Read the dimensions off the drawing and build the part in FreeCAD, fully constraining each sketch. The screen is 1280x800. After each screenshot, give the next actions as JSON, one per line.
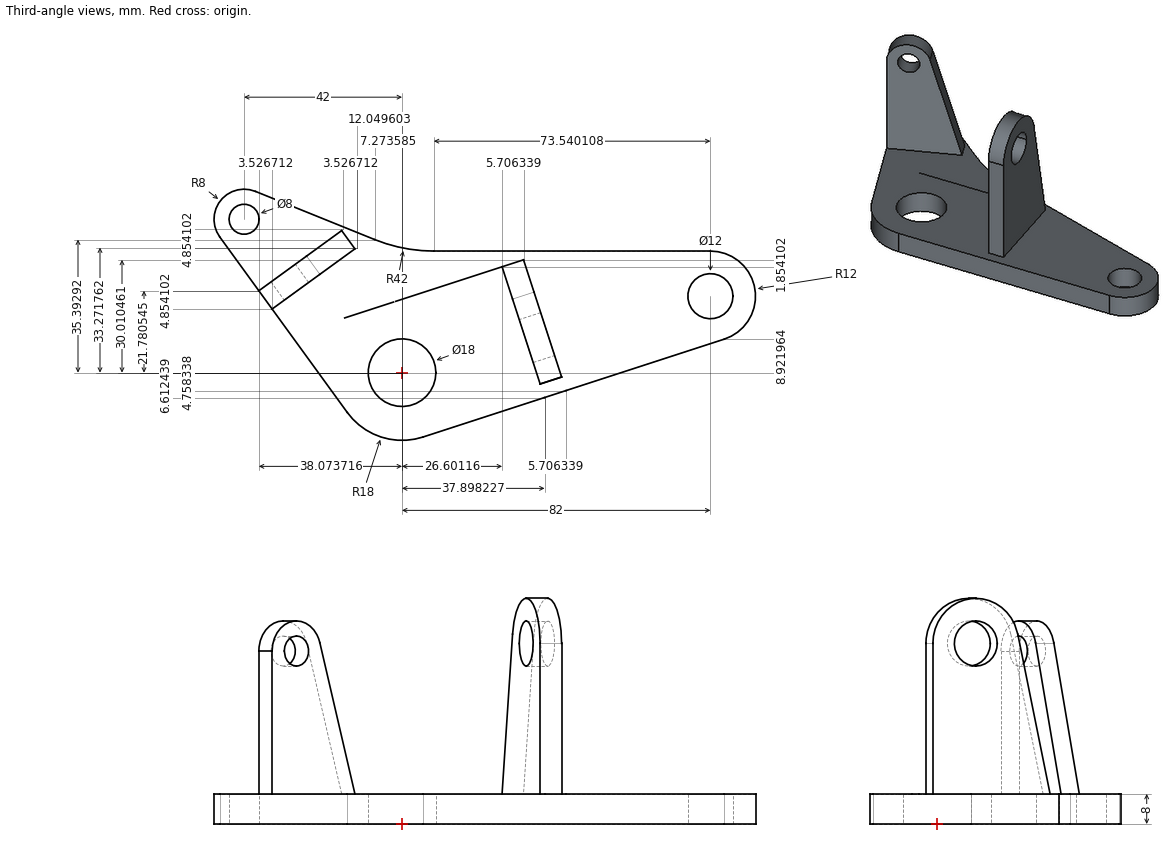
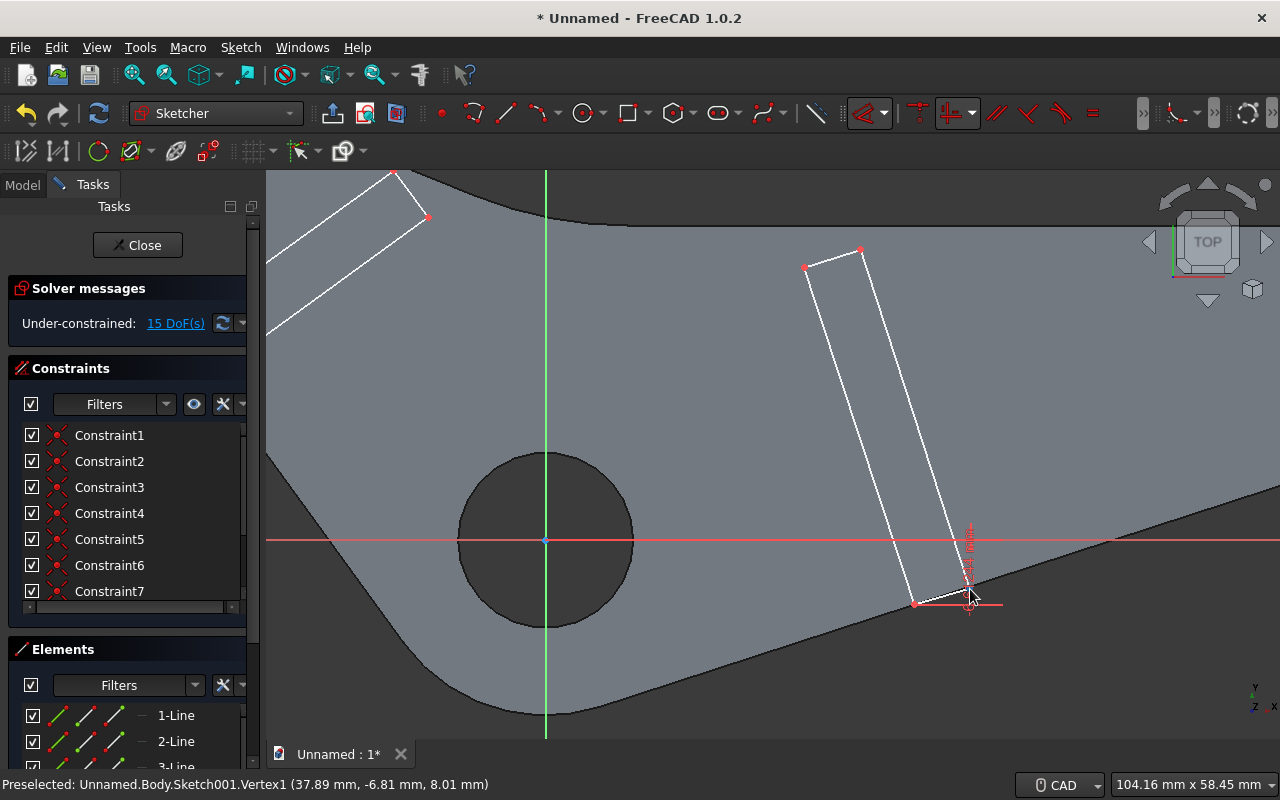
{"action": "left_click", "coordinate": [970, 589]}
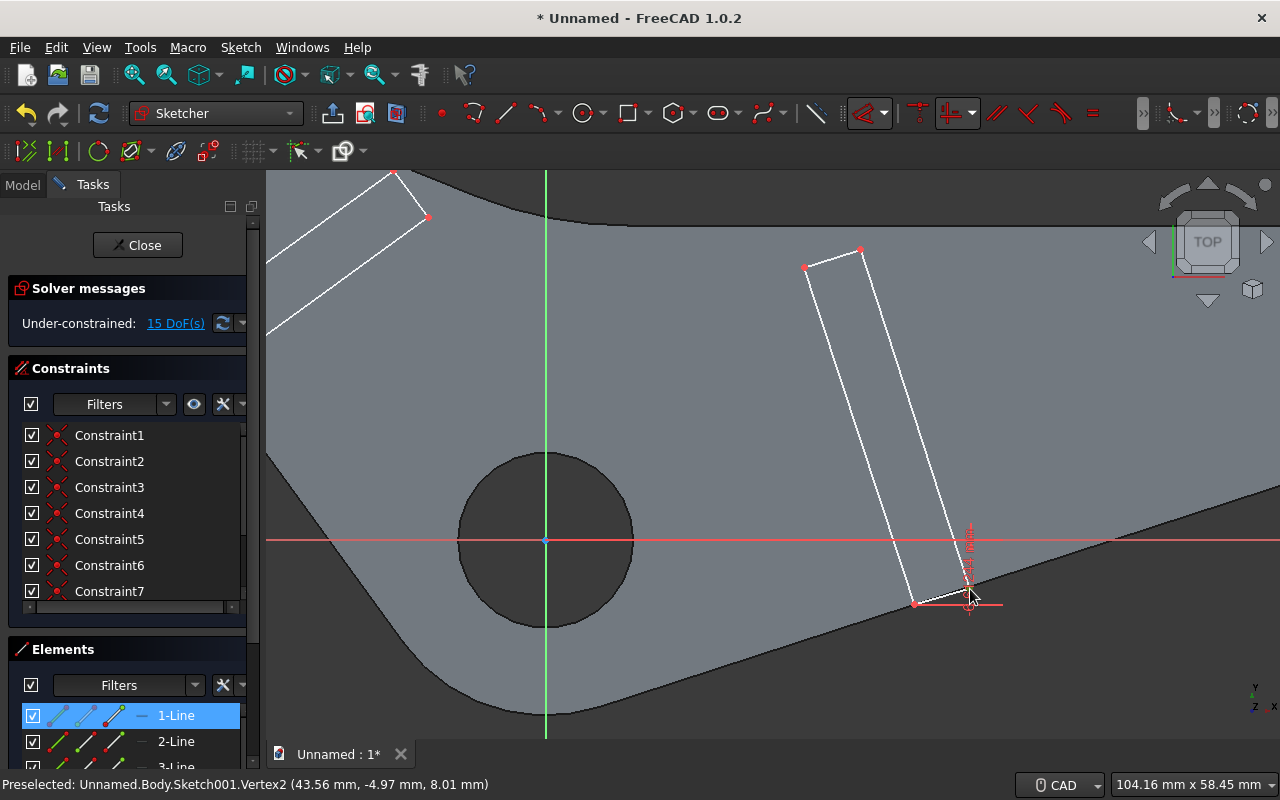
{"action": "left_click", "coordinate": [886, 114]}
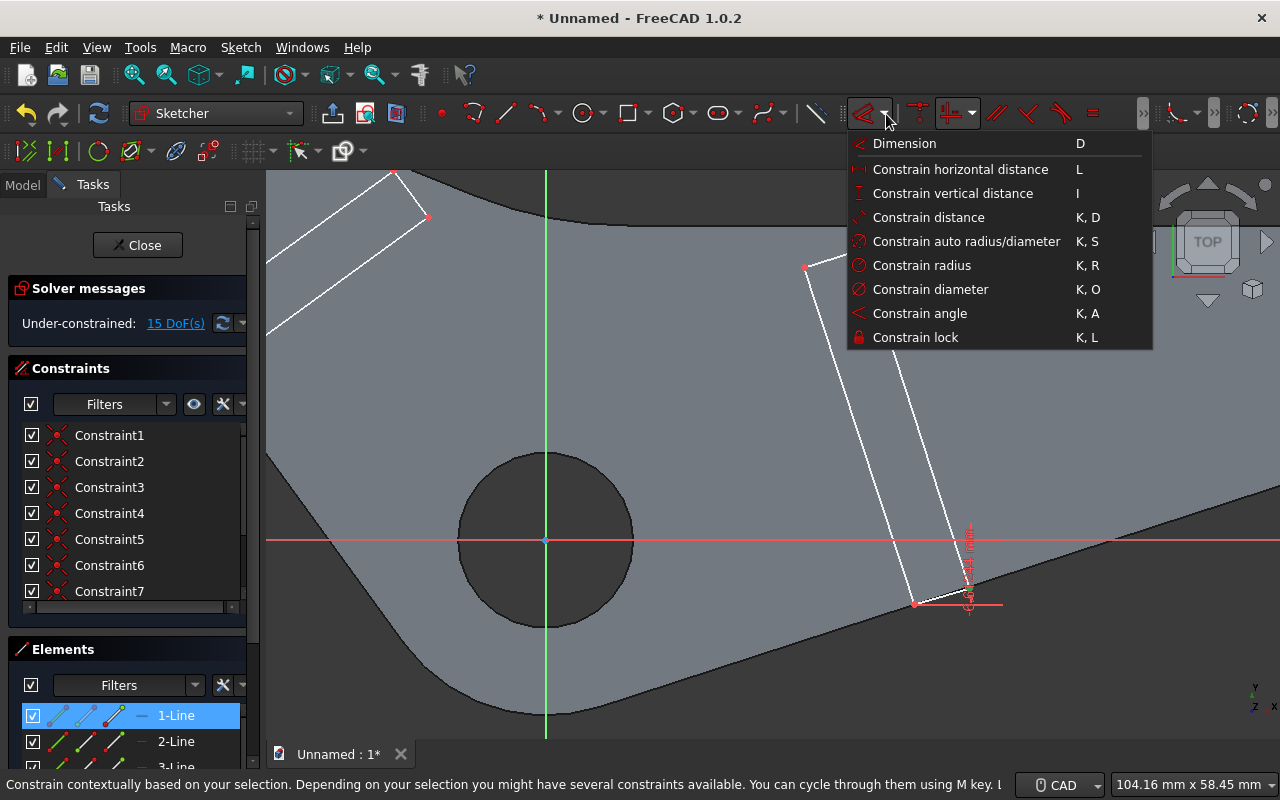
{"action": "left_click", "coordinate": [1000, 193]}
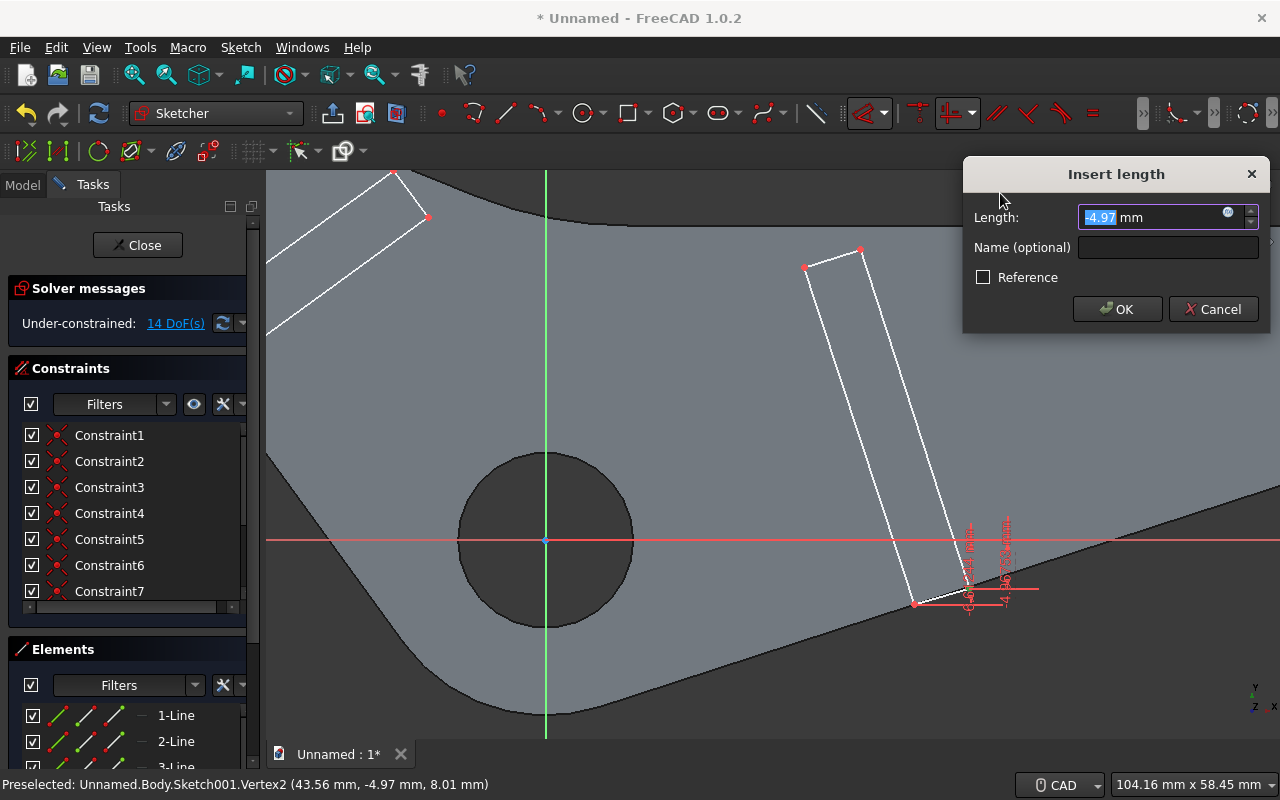
{"action": "type", "text": "-4.758338"}
{"action": "key", "text": "Return"}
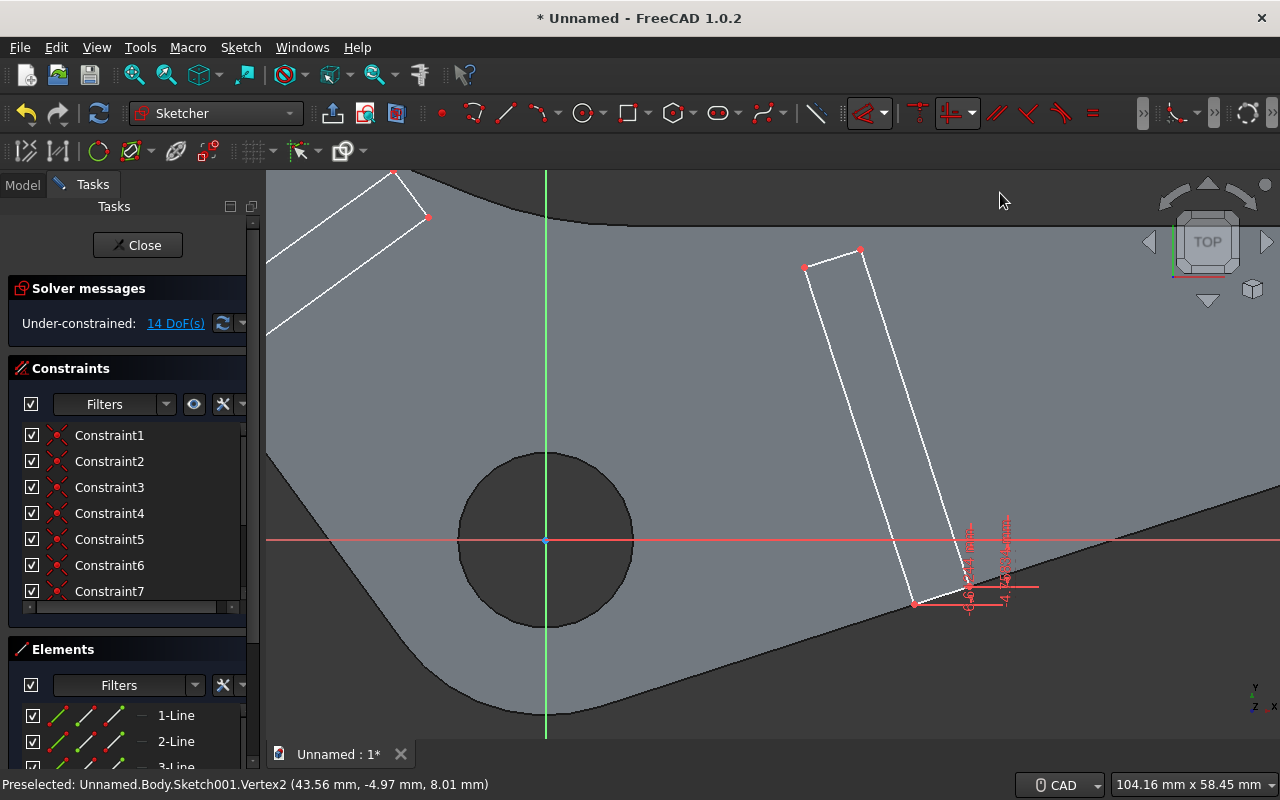
{"action": "left_click", "coordinate": [804, 268]}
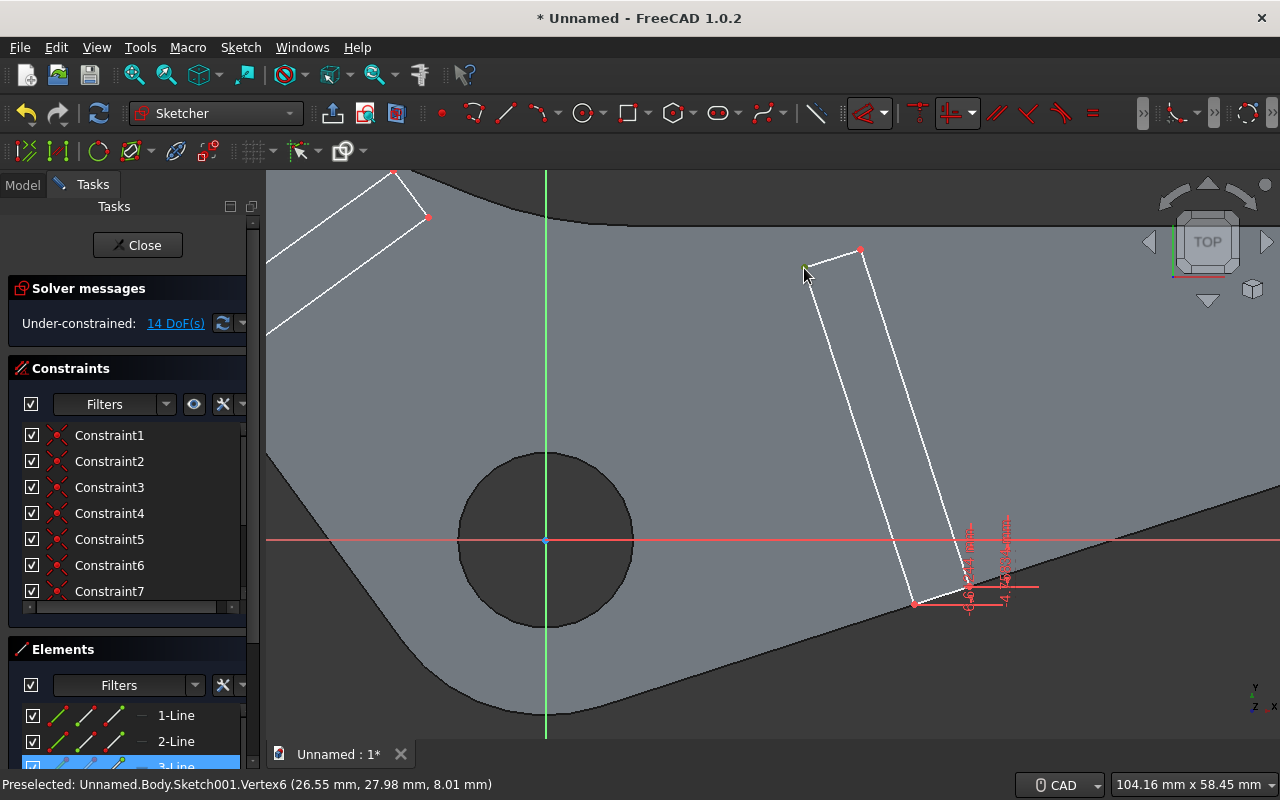
{"action": "key", "text": "l"}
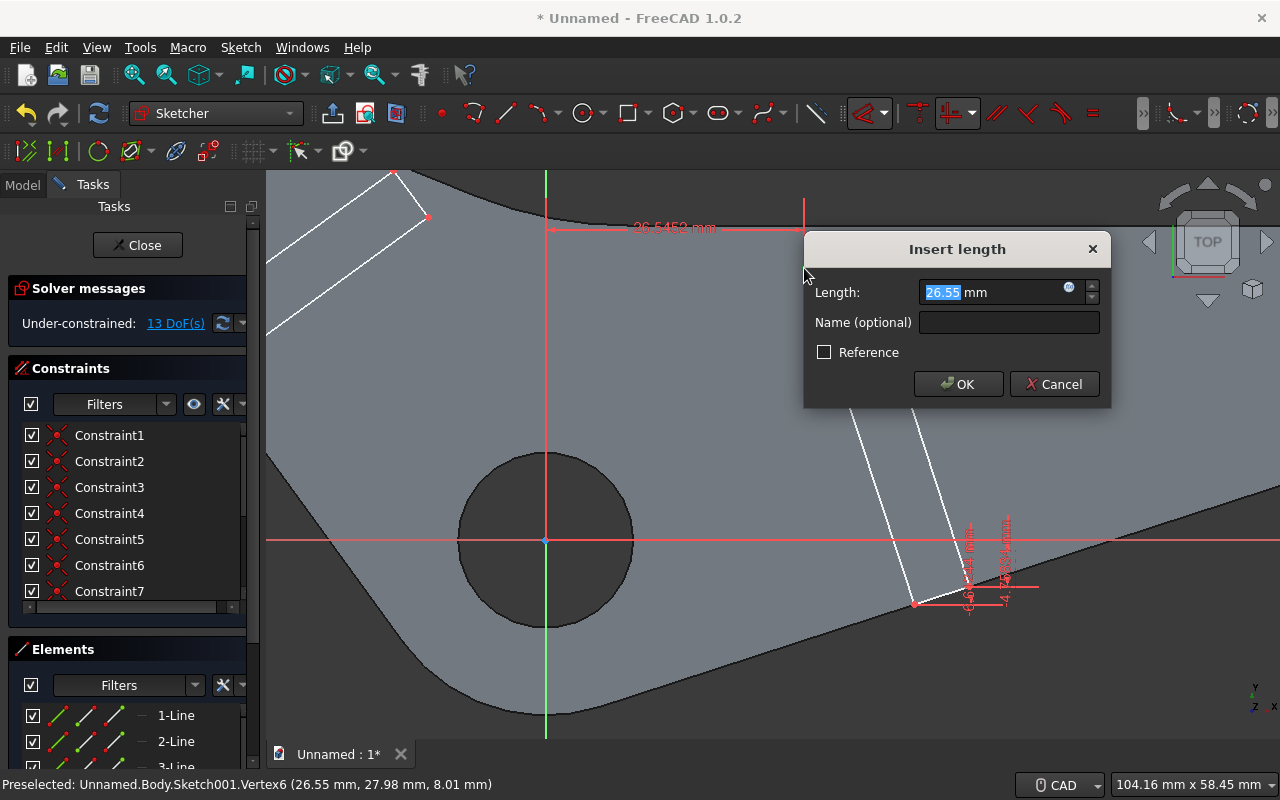
{"action": "type", "text": "26.60116"}
{"action": "key", "text": "Return"}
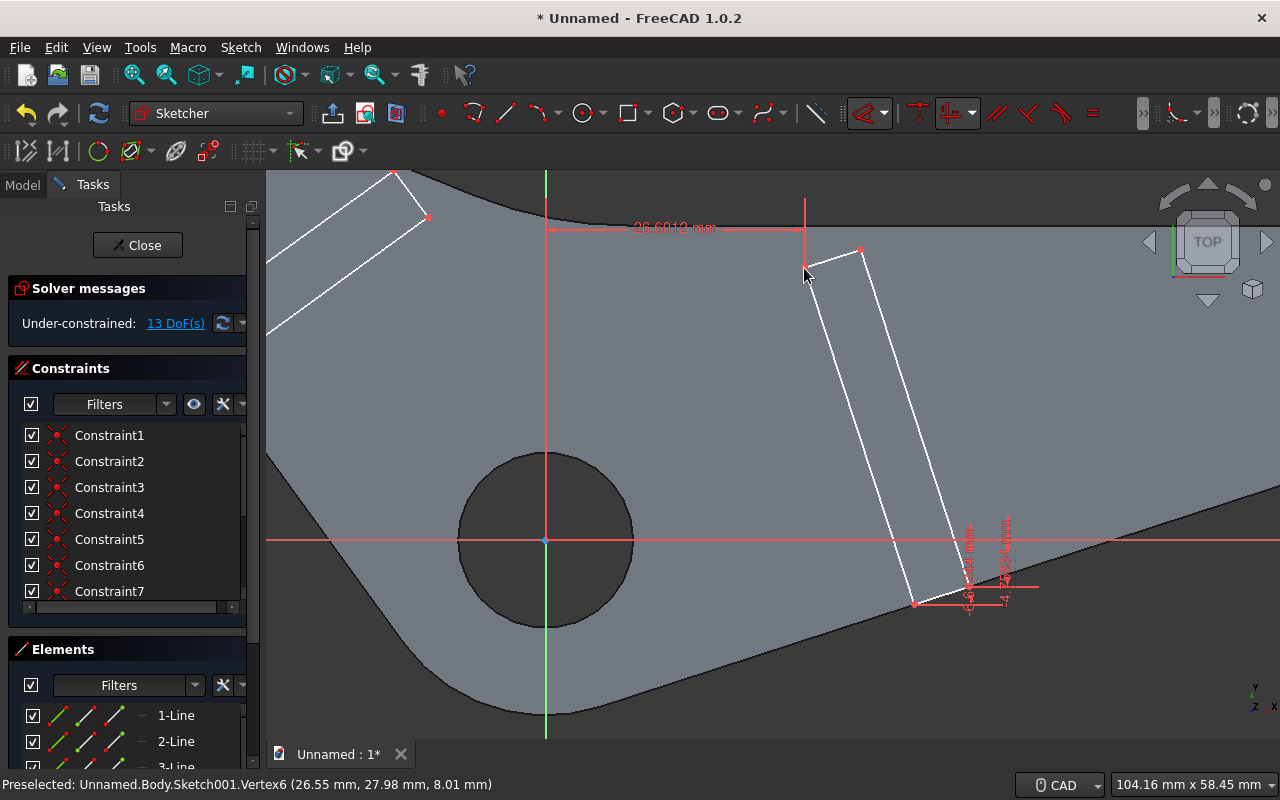
{"action": "left_click", "coordinate": [931, 599]}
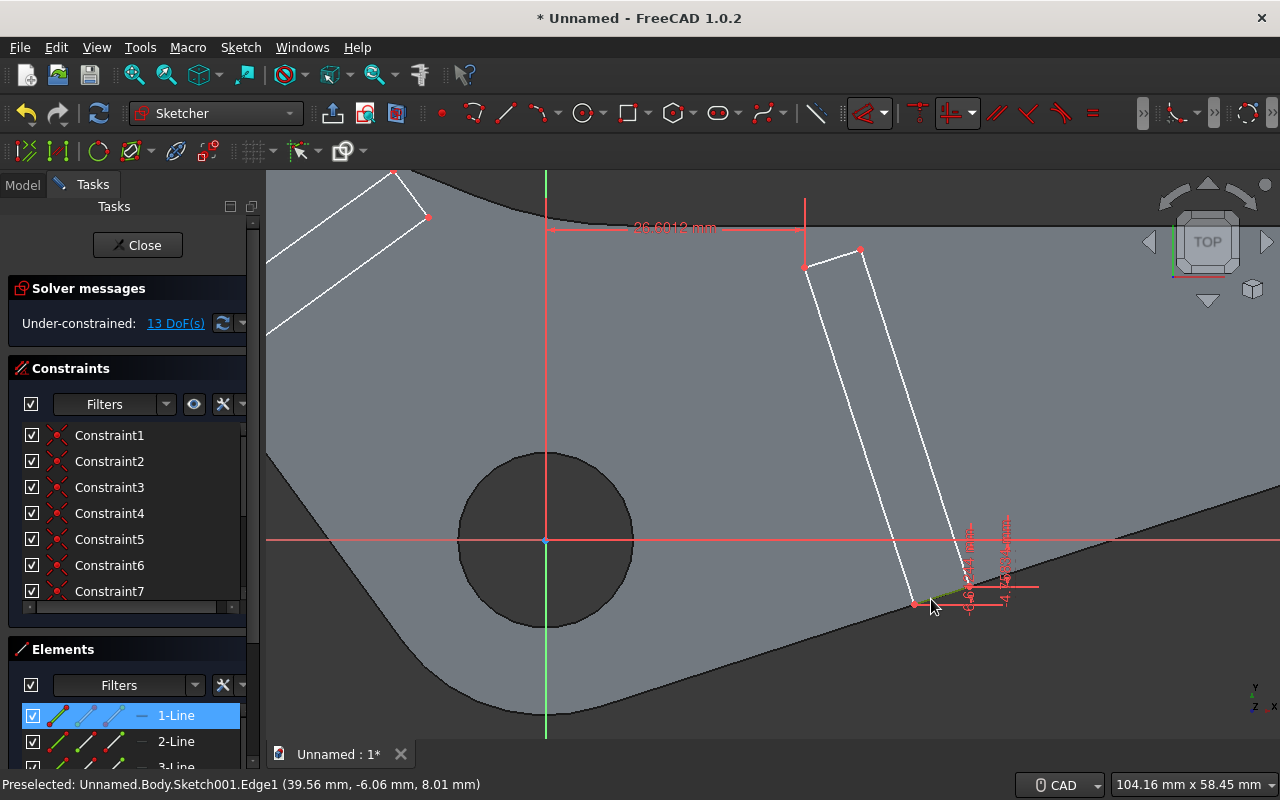
{"action": "key", "text": "l"}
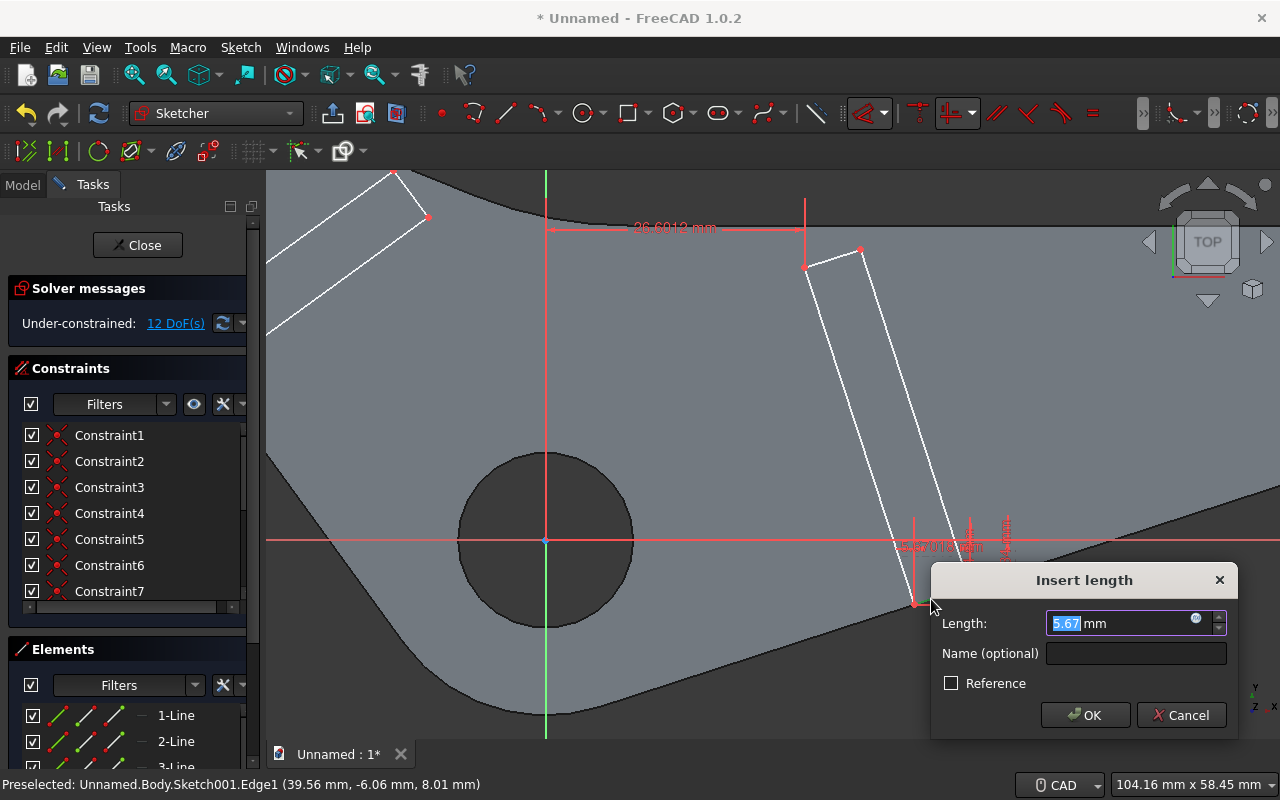
{"action": "type", "text": "5.706339"}
{"action": "key", "text": "Return"}